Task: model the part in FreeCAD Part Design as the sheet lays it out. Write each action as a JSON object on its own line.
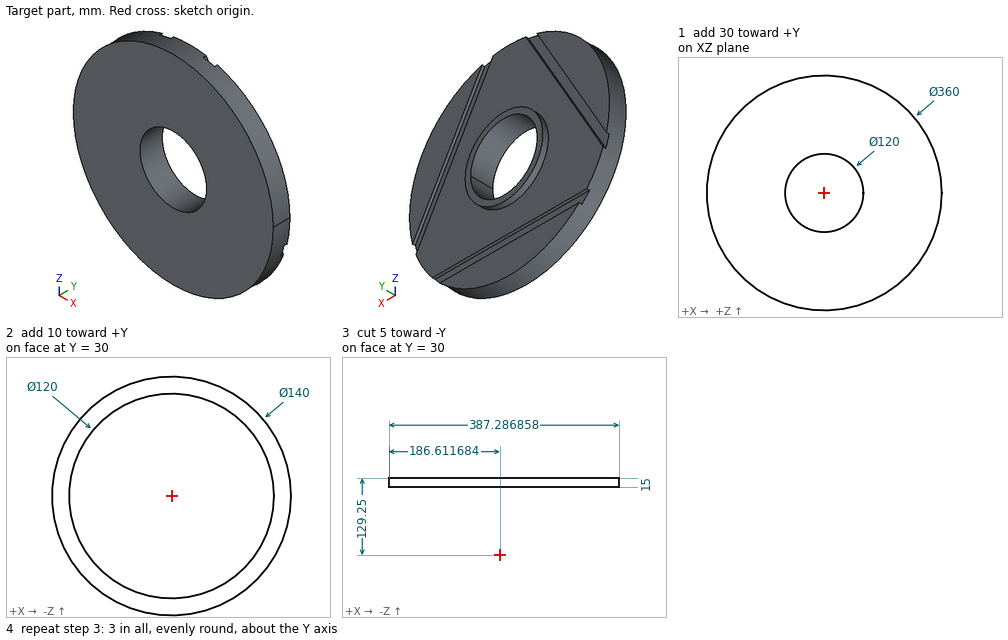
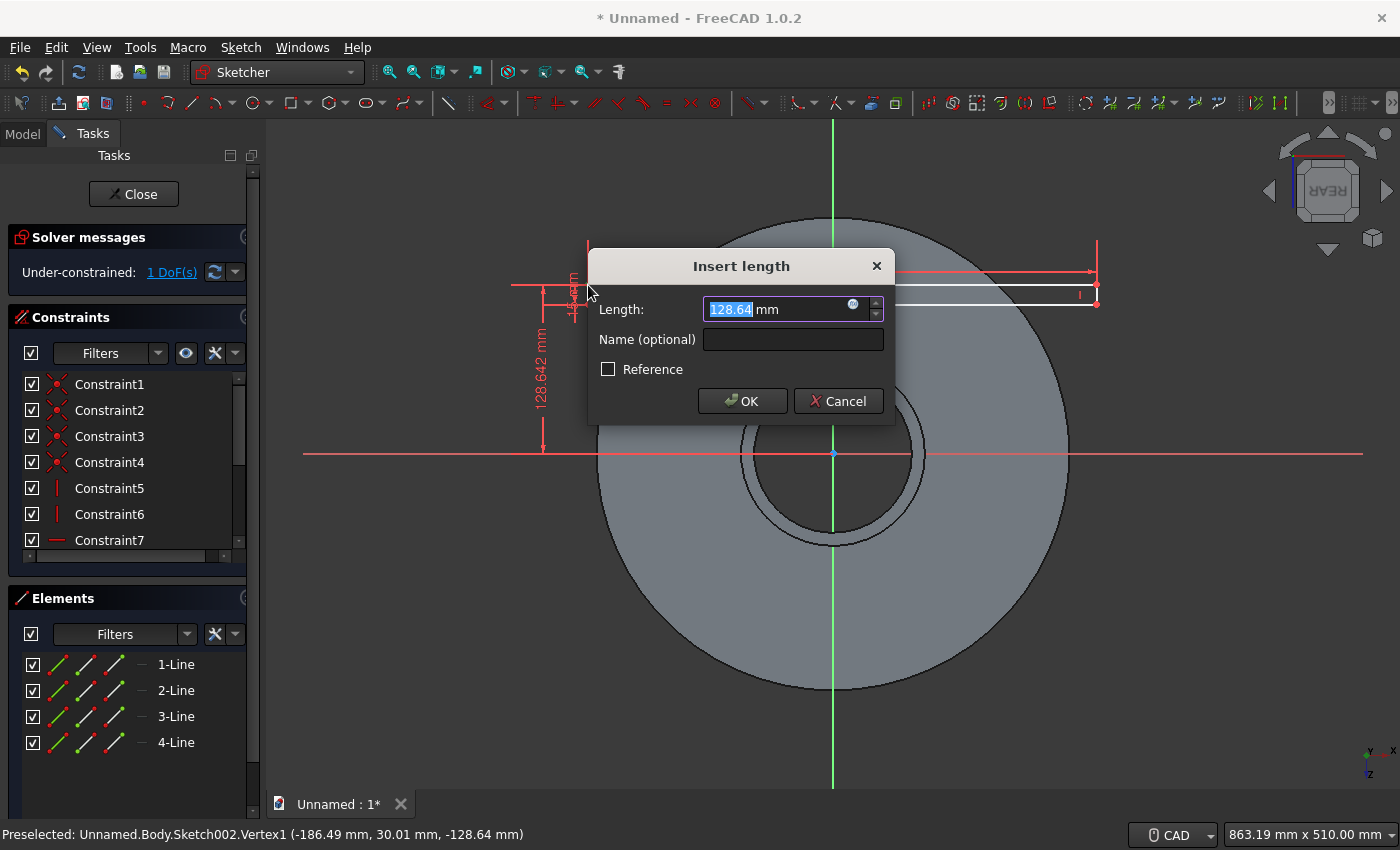
{"action": "type", "text": "129.25"}
{"action": "key", "text": "Return"}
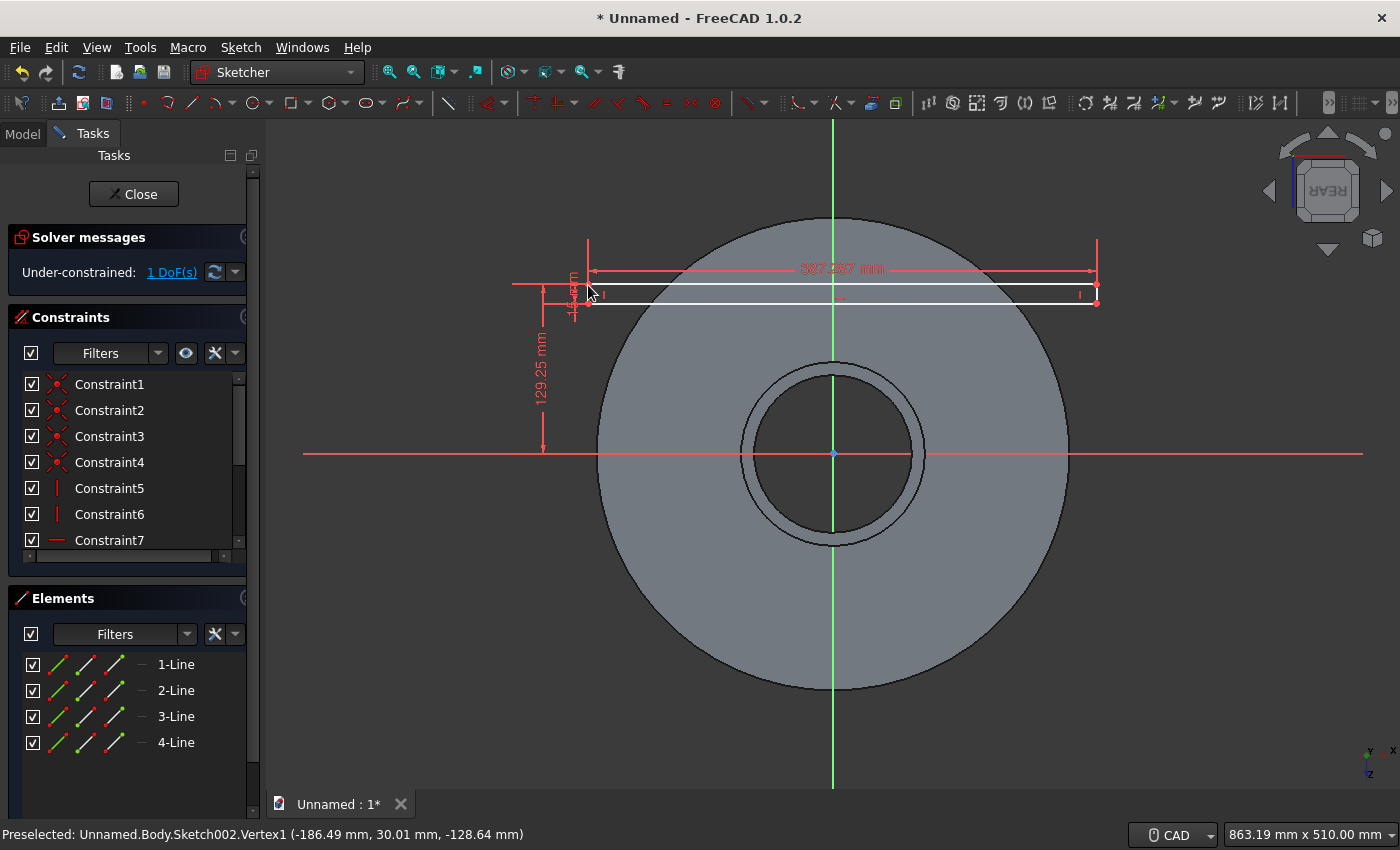
{"action": "left_click", "coordinate": [588, 284]}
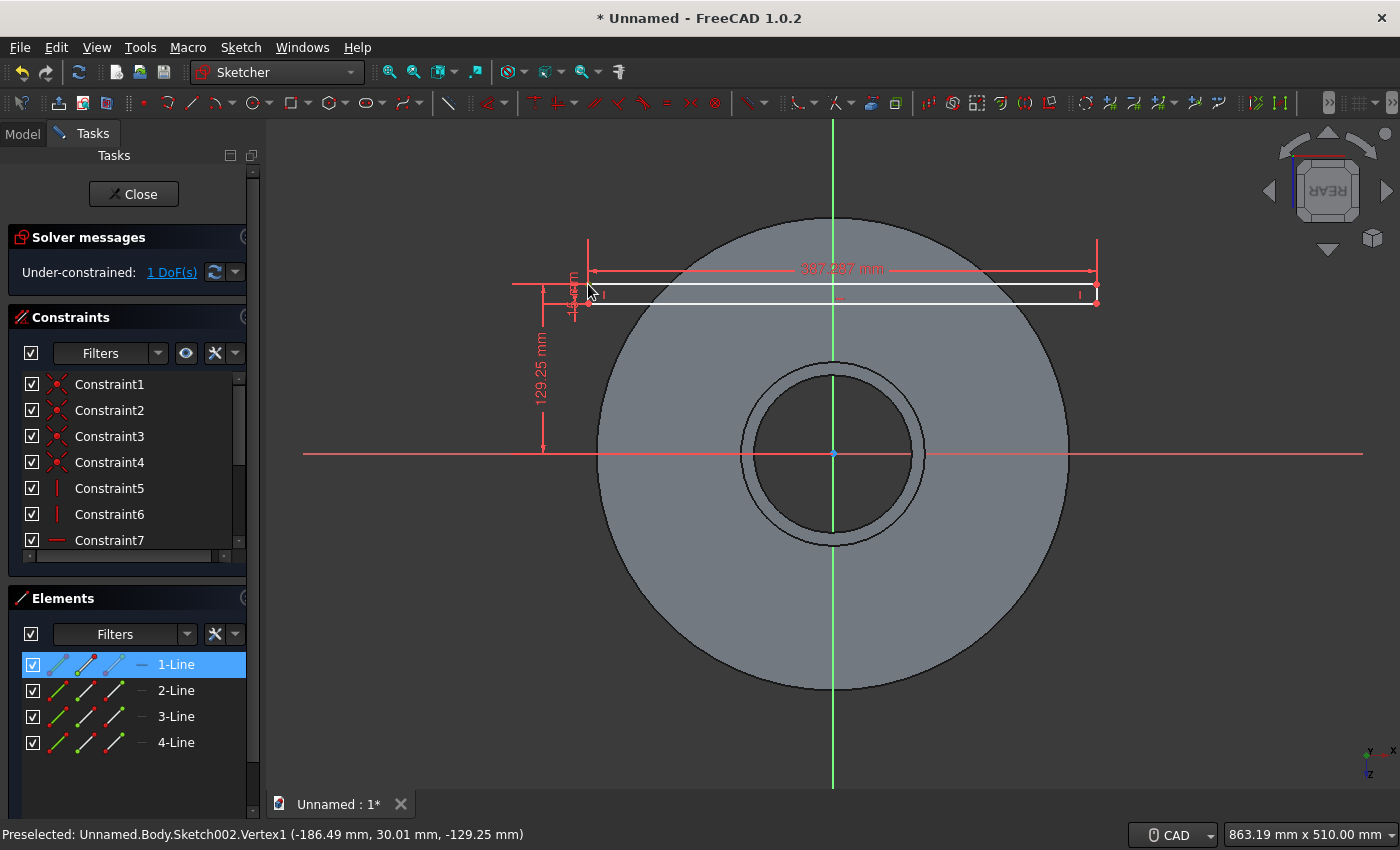
{"action": "key", "text": "l"}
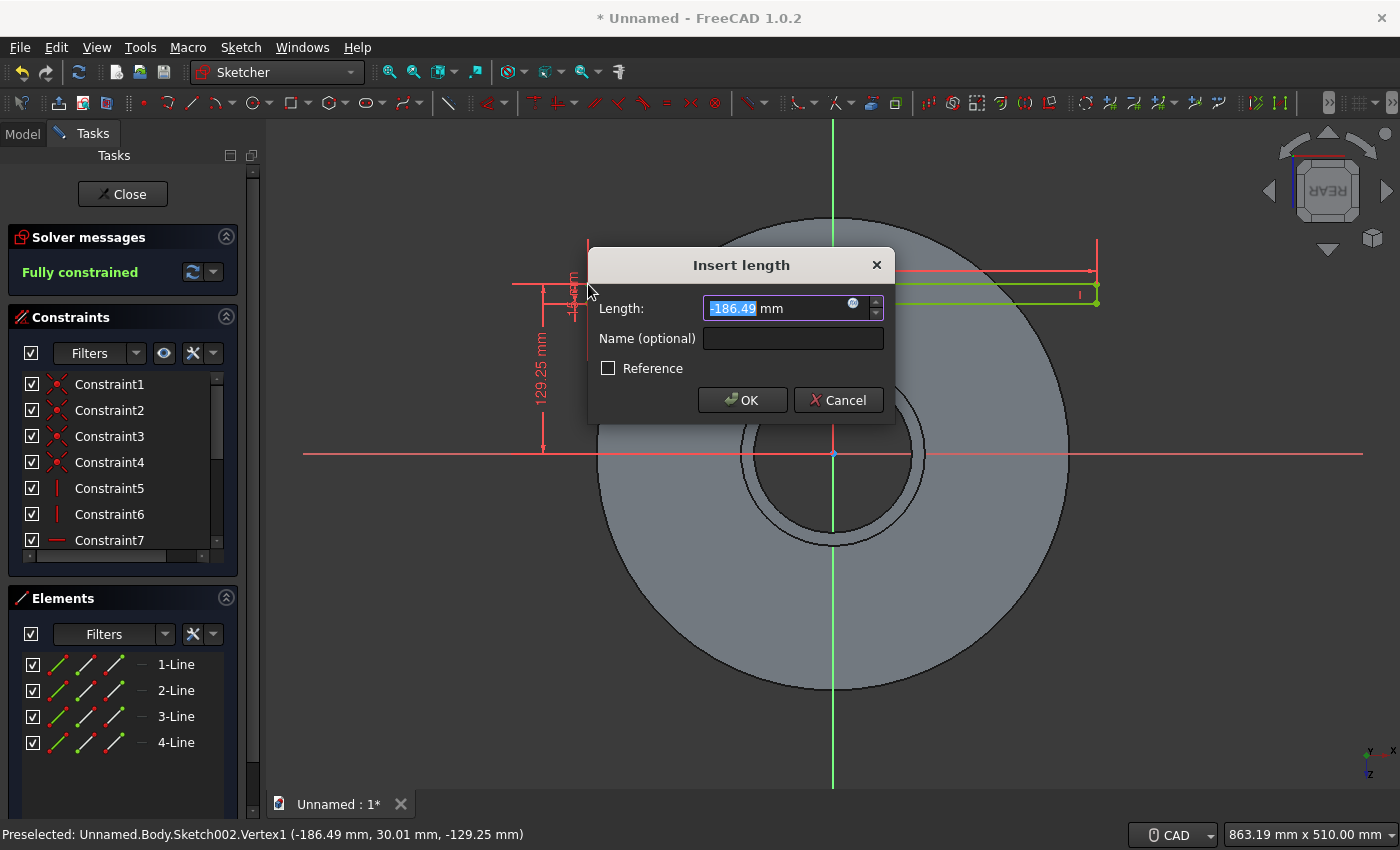
{"action": "type", "text": "-186.611684"}
{"action": "key", "text": "Return"}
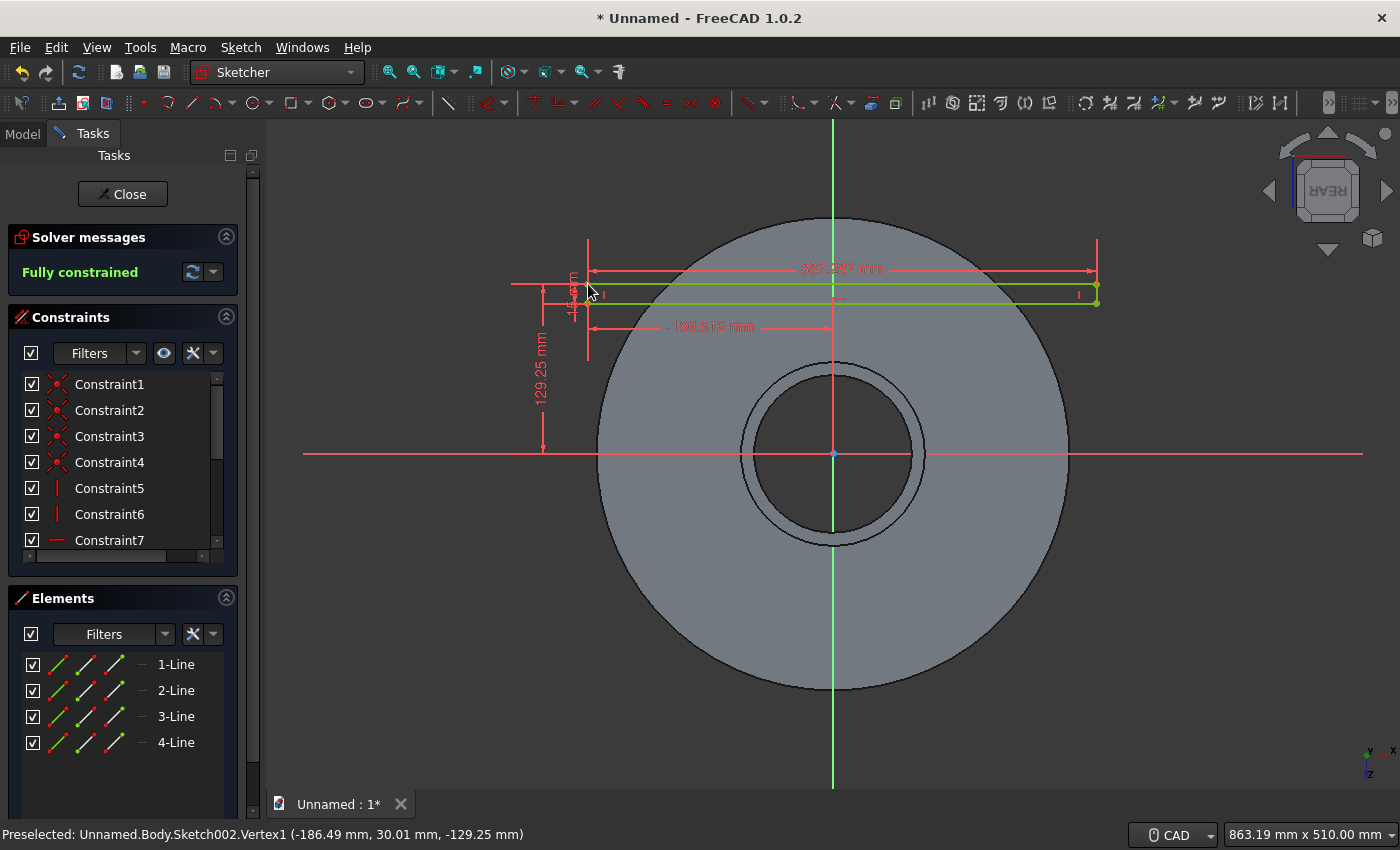
{"action": "left_click", "coordinate": [123, 194]}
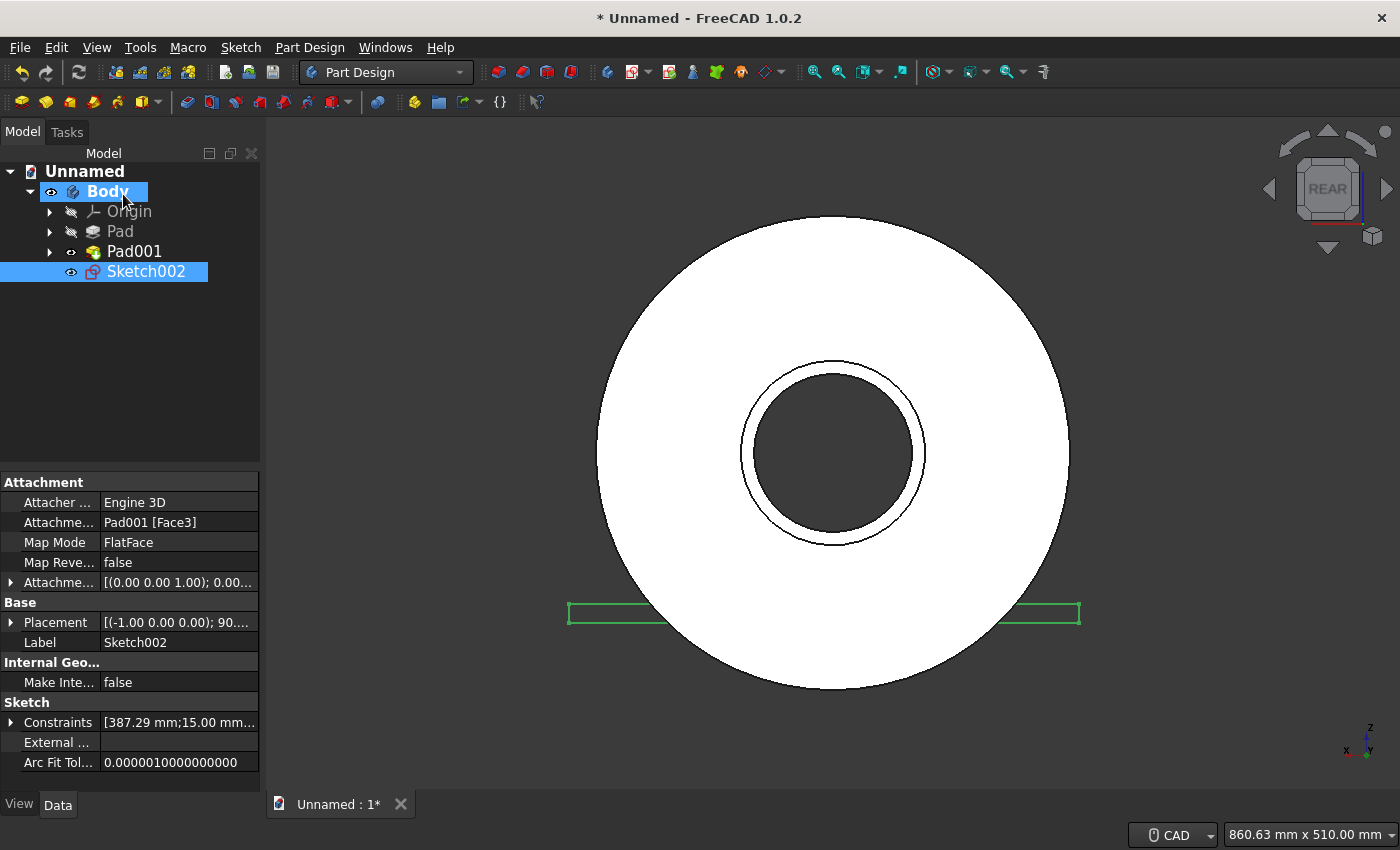
{"action": "left_click", "coordinate": [188, 102]}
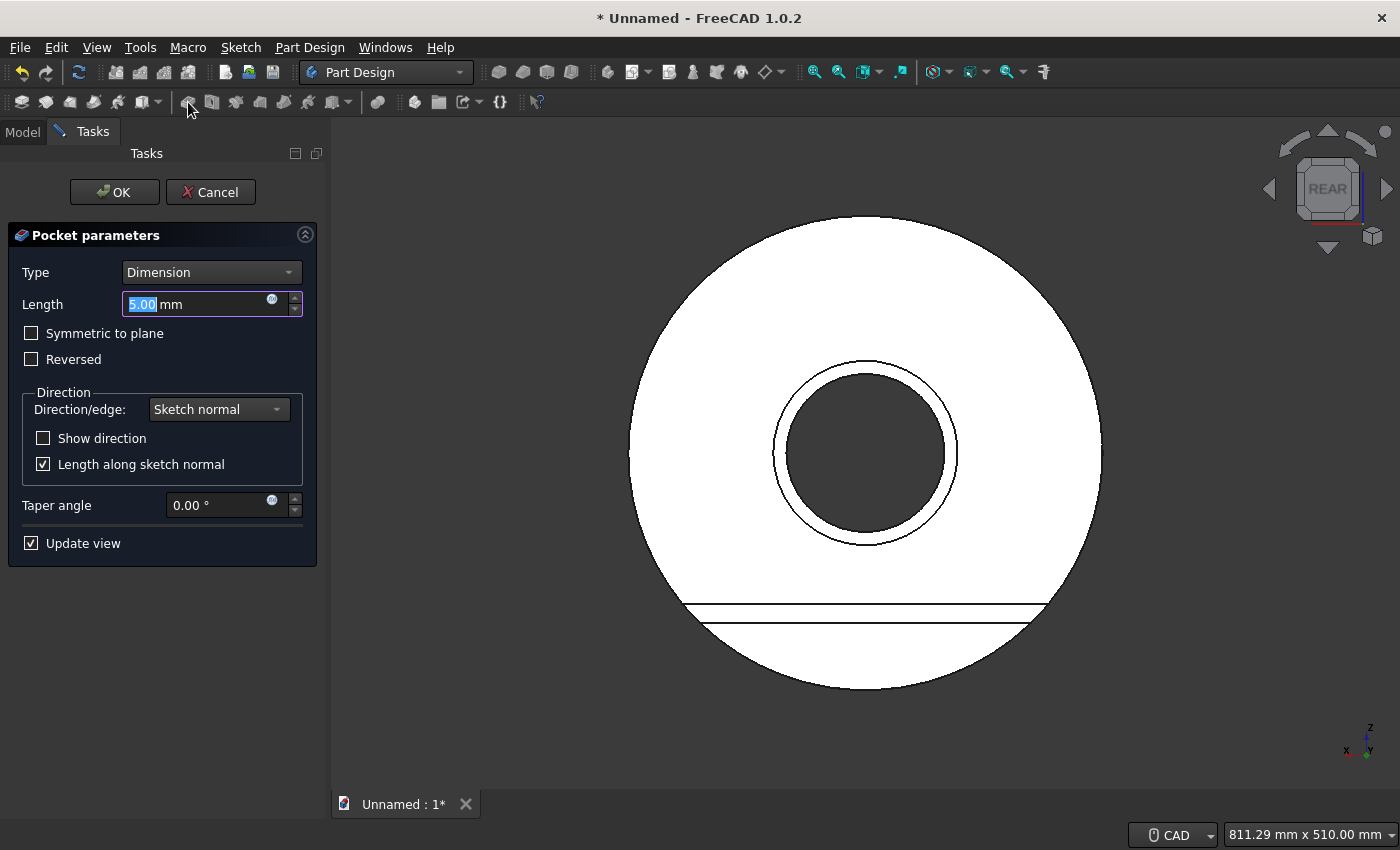
{"action": "type", "text": "5"}
{"action": "key", "text": "Tab"}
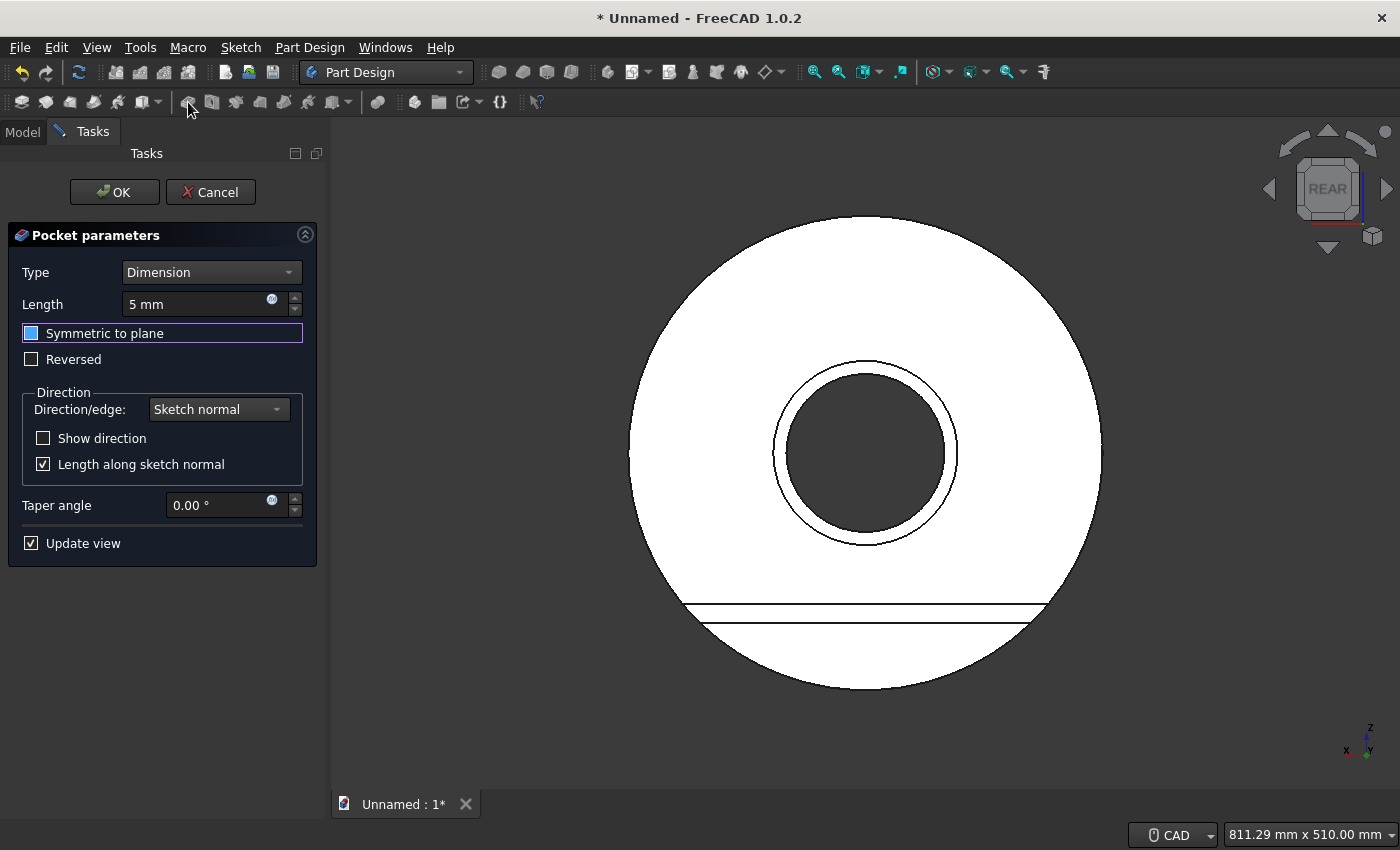
{"action": "left_click", "coordinate": [115, 192]}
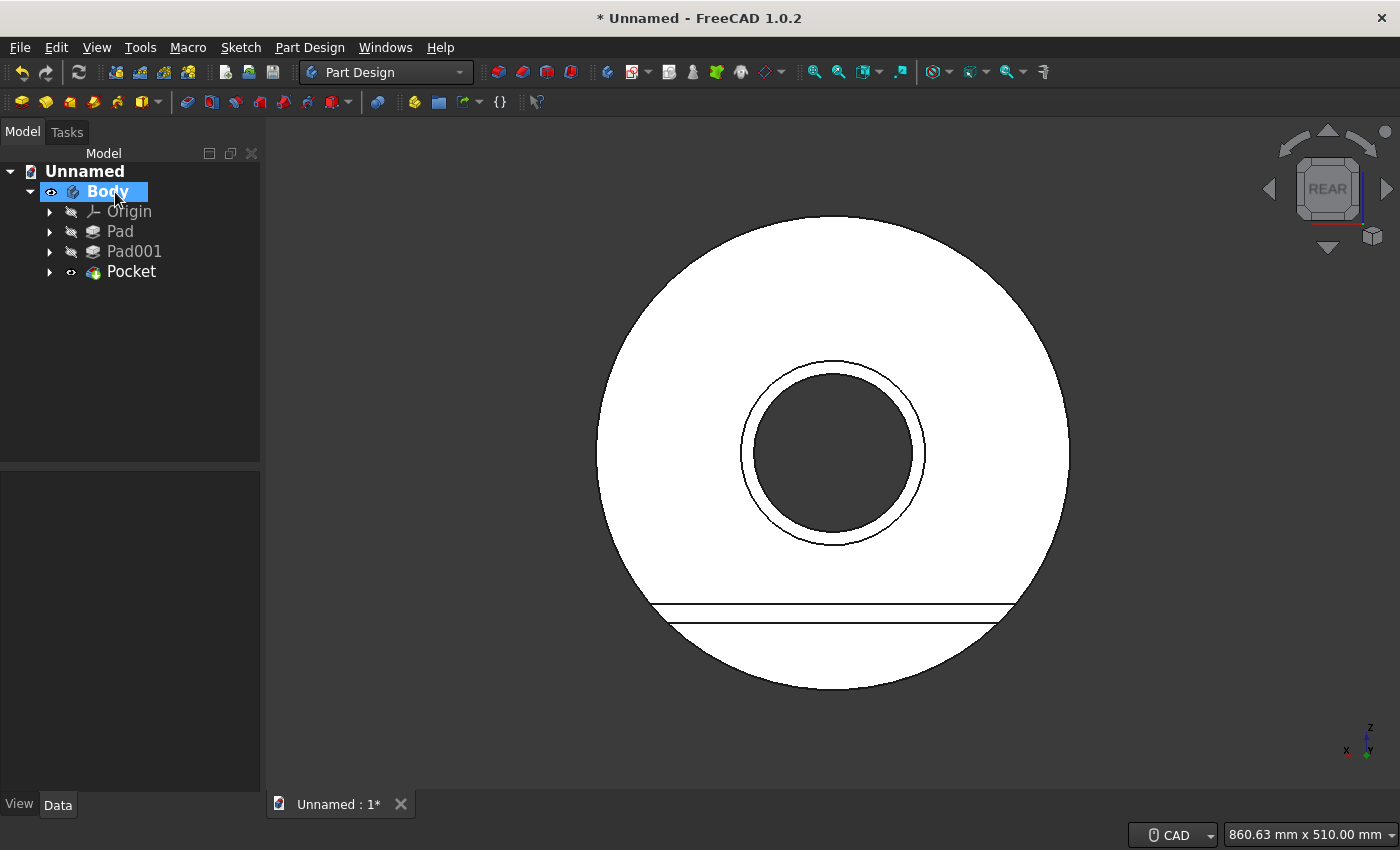
{"action": "left_click", "coordinate": [116, 272]}